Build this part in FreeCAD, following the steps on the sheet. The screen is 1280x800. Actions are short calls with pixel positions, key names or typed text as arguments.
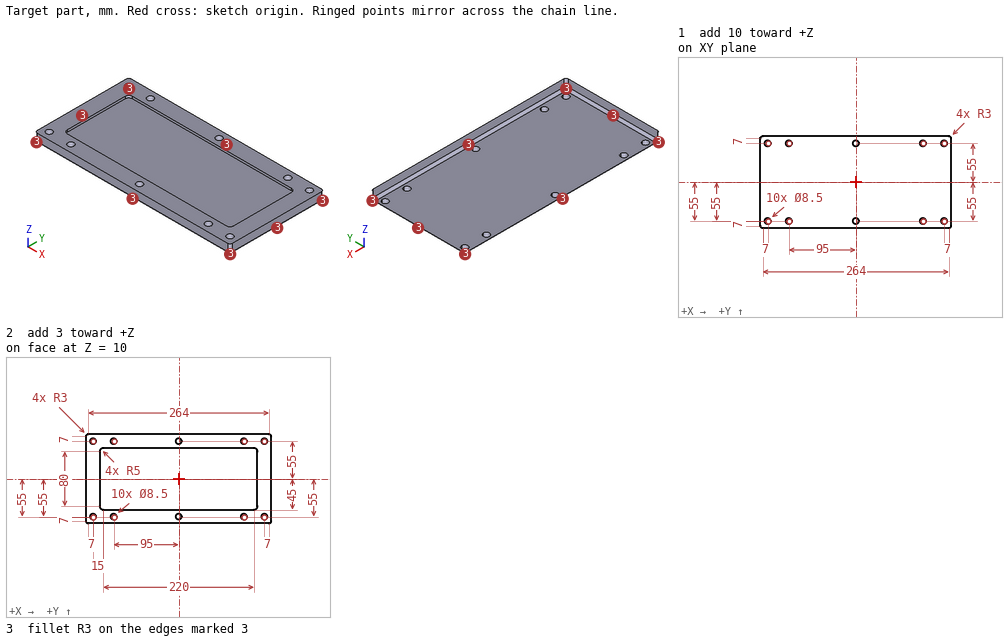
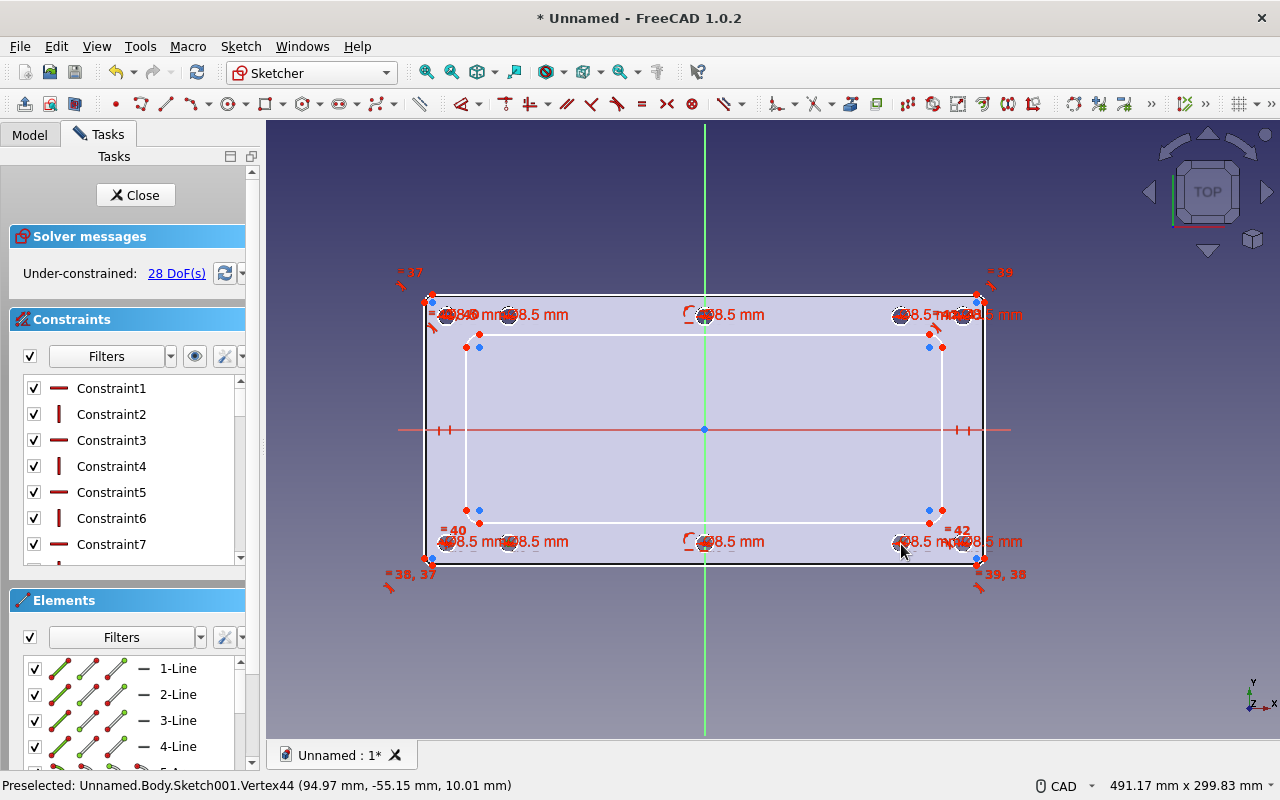
click(705, 671)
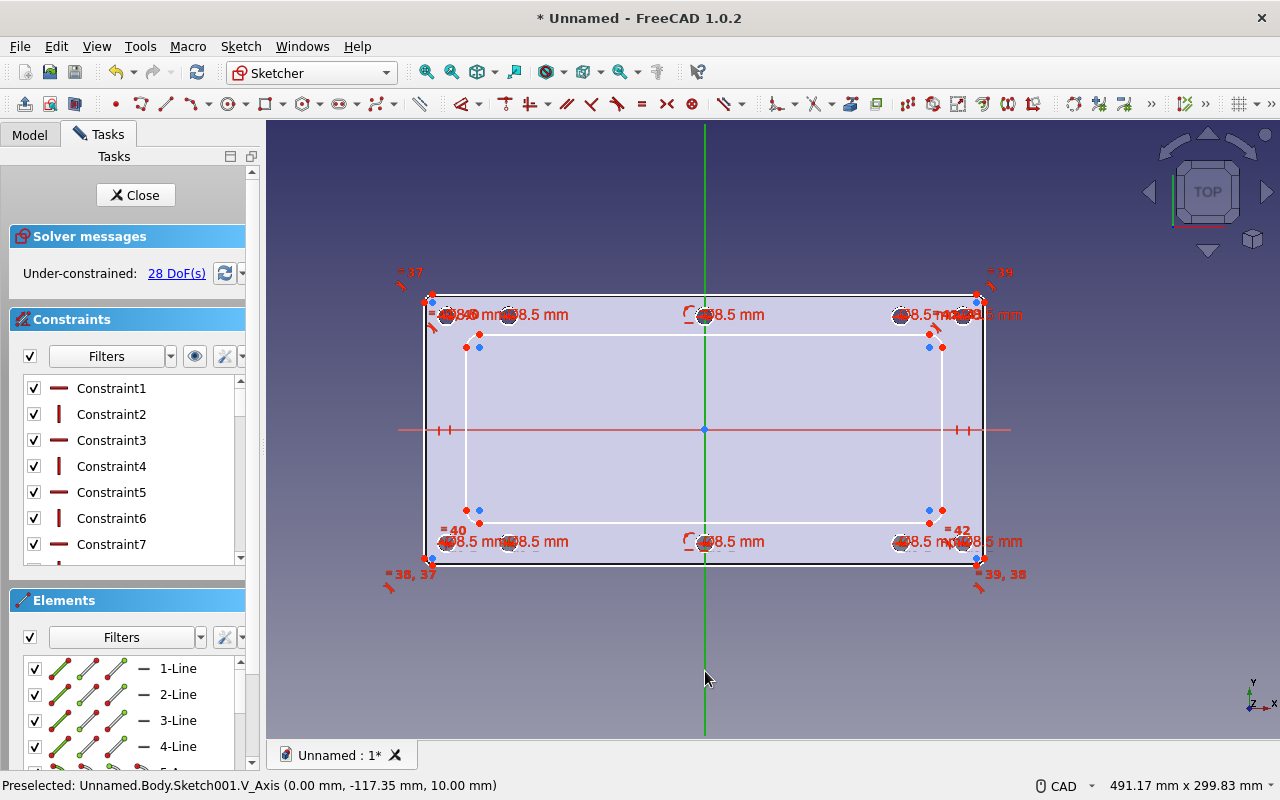
click(667, 104)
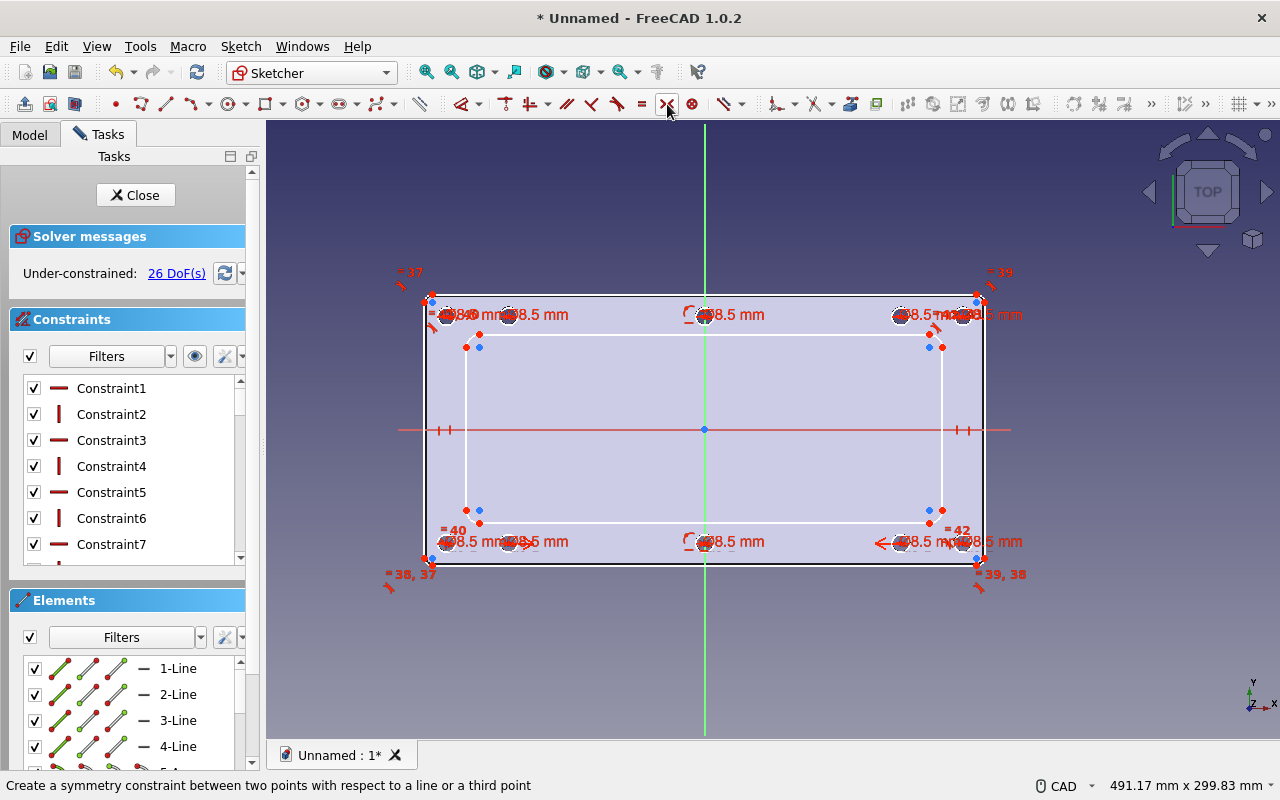
click(447, 544)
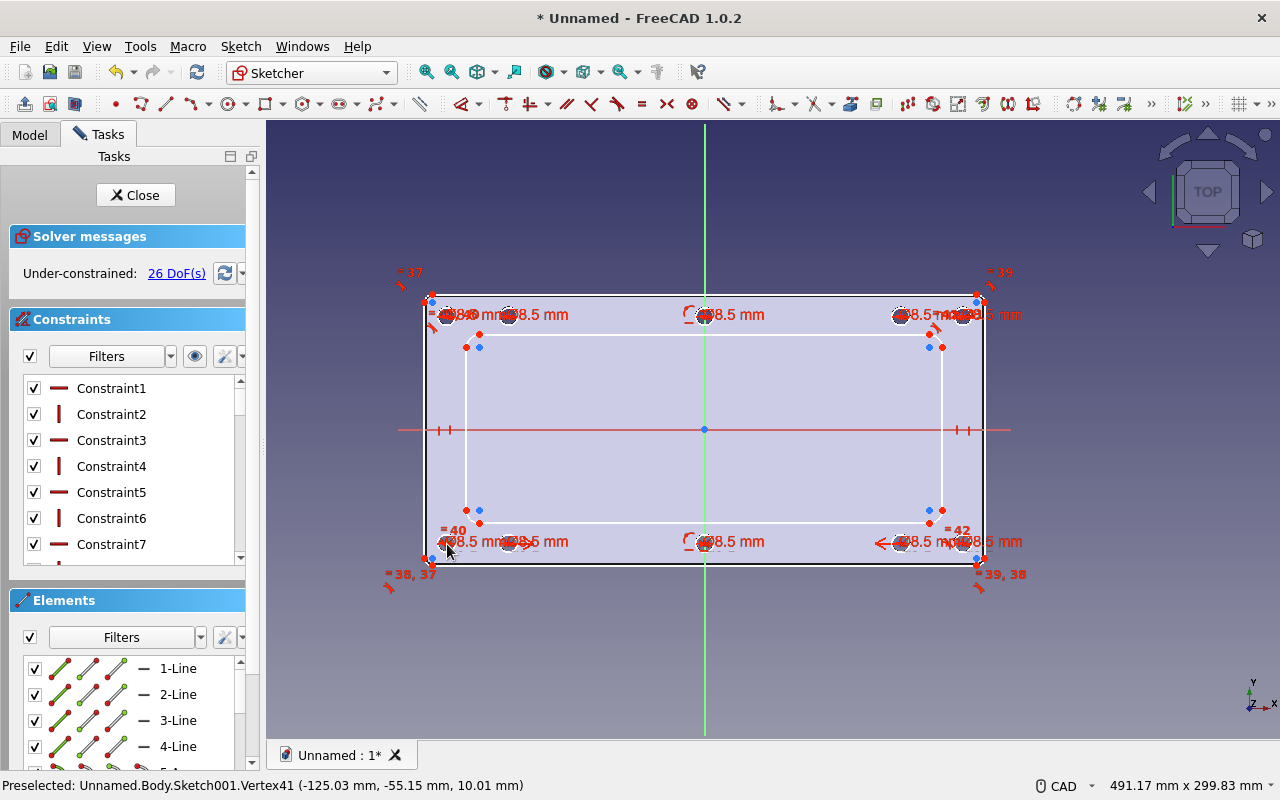
scroll(963, 544, up, 4)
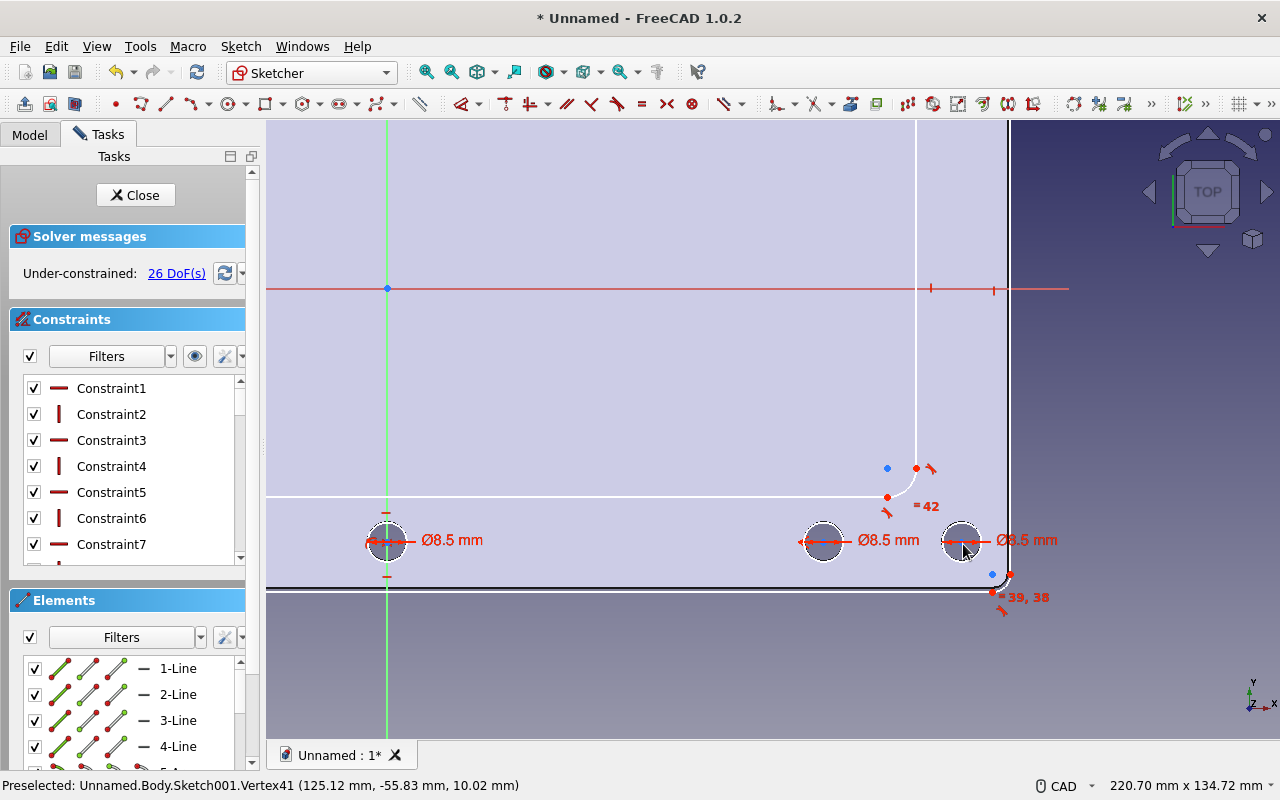
click(962, 542)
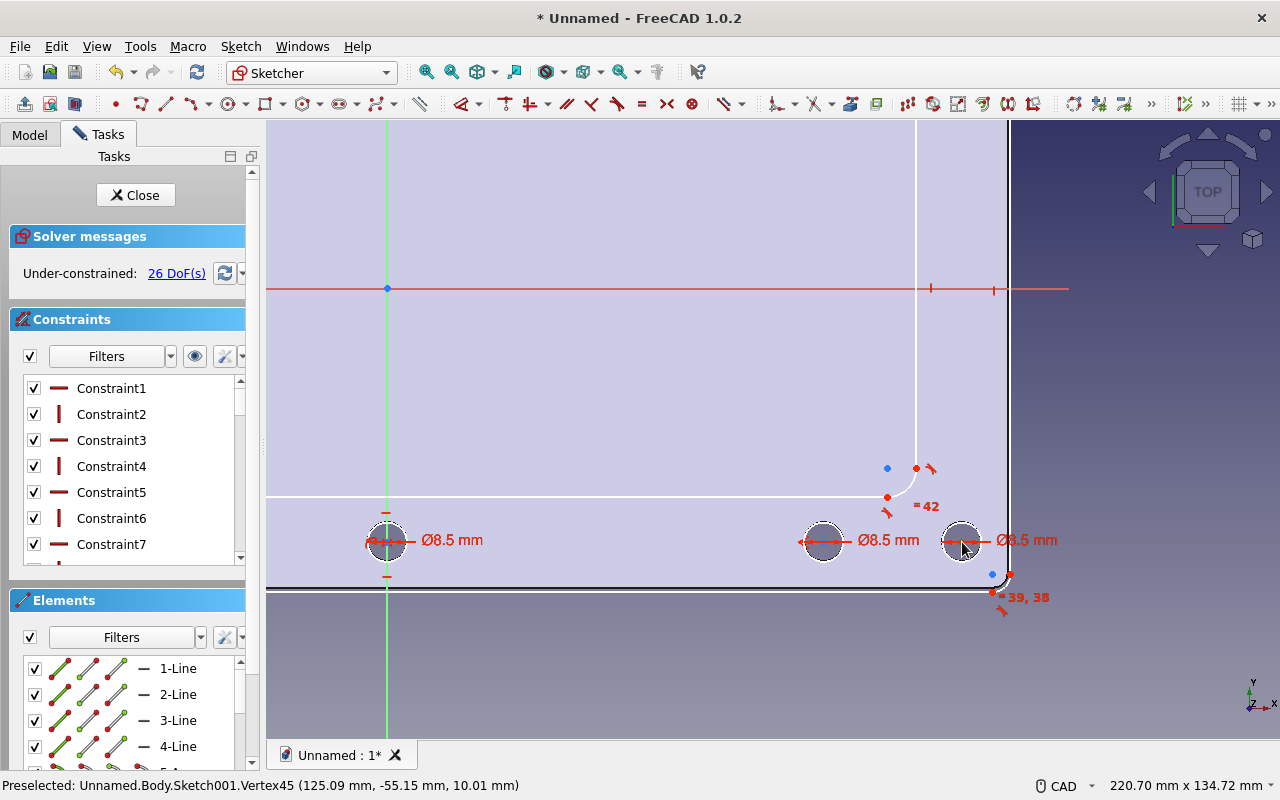
click(387, 671)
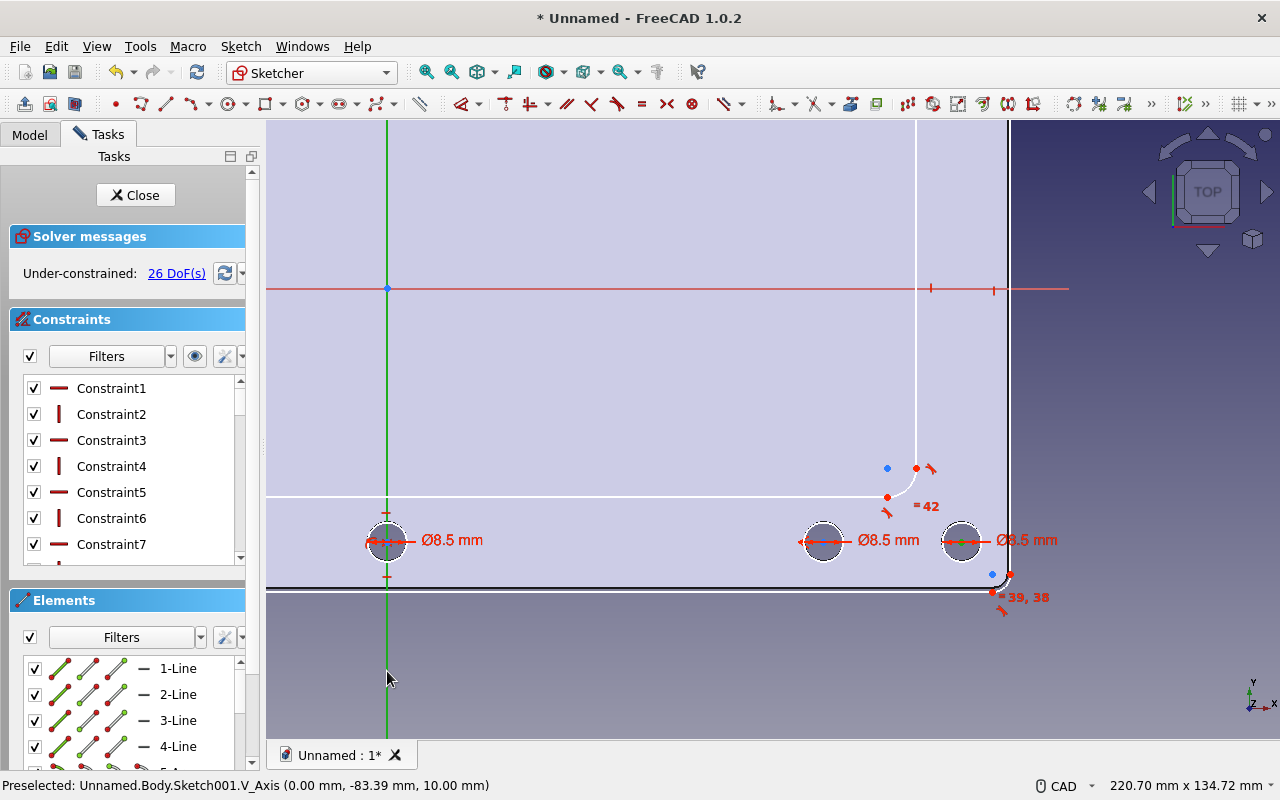
click(667, 104)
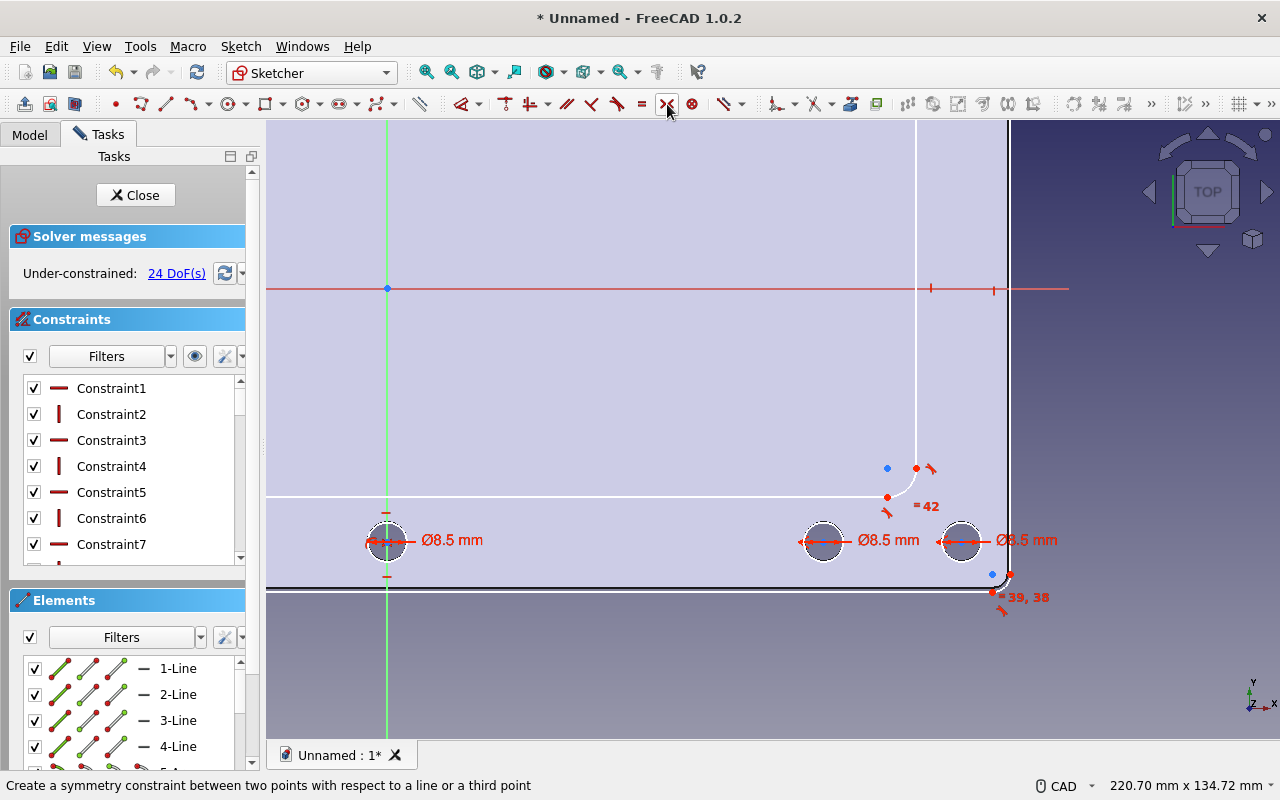
scroll(963, 544, down, 4)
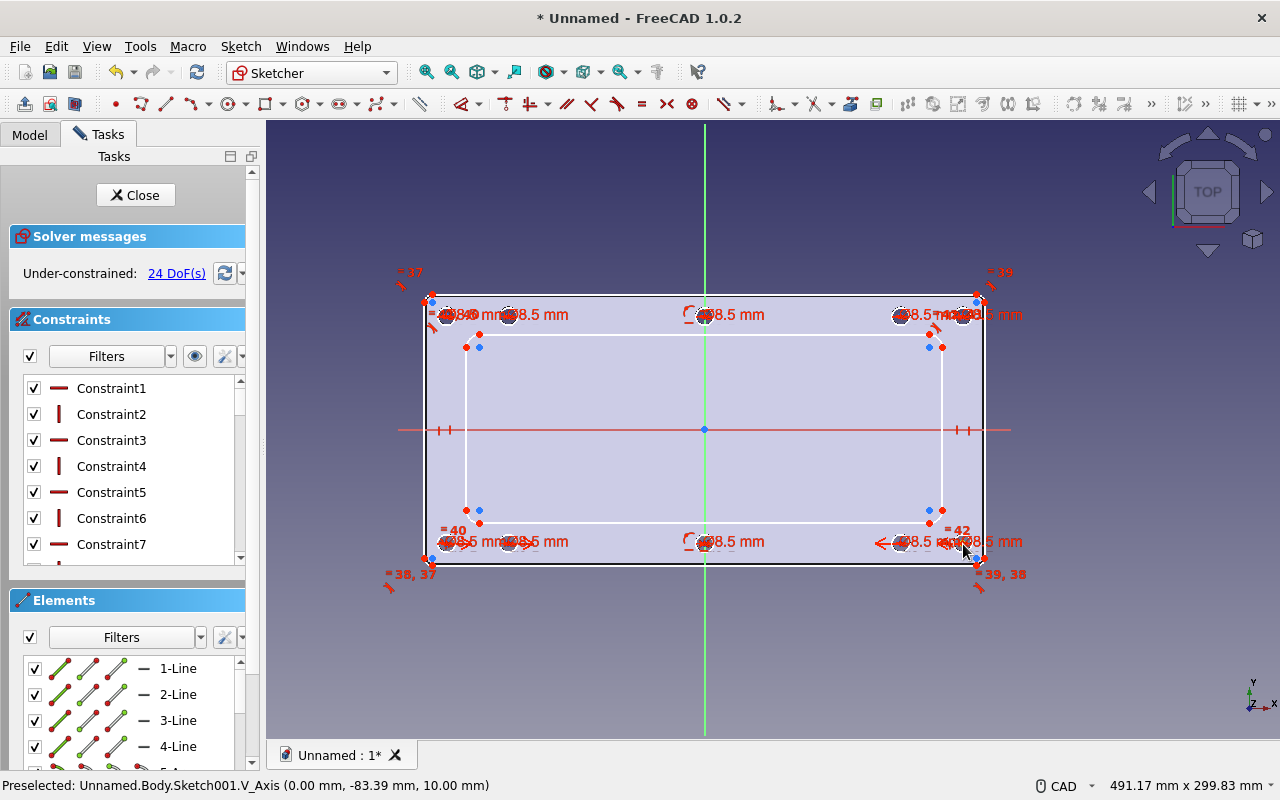
click(447, 544)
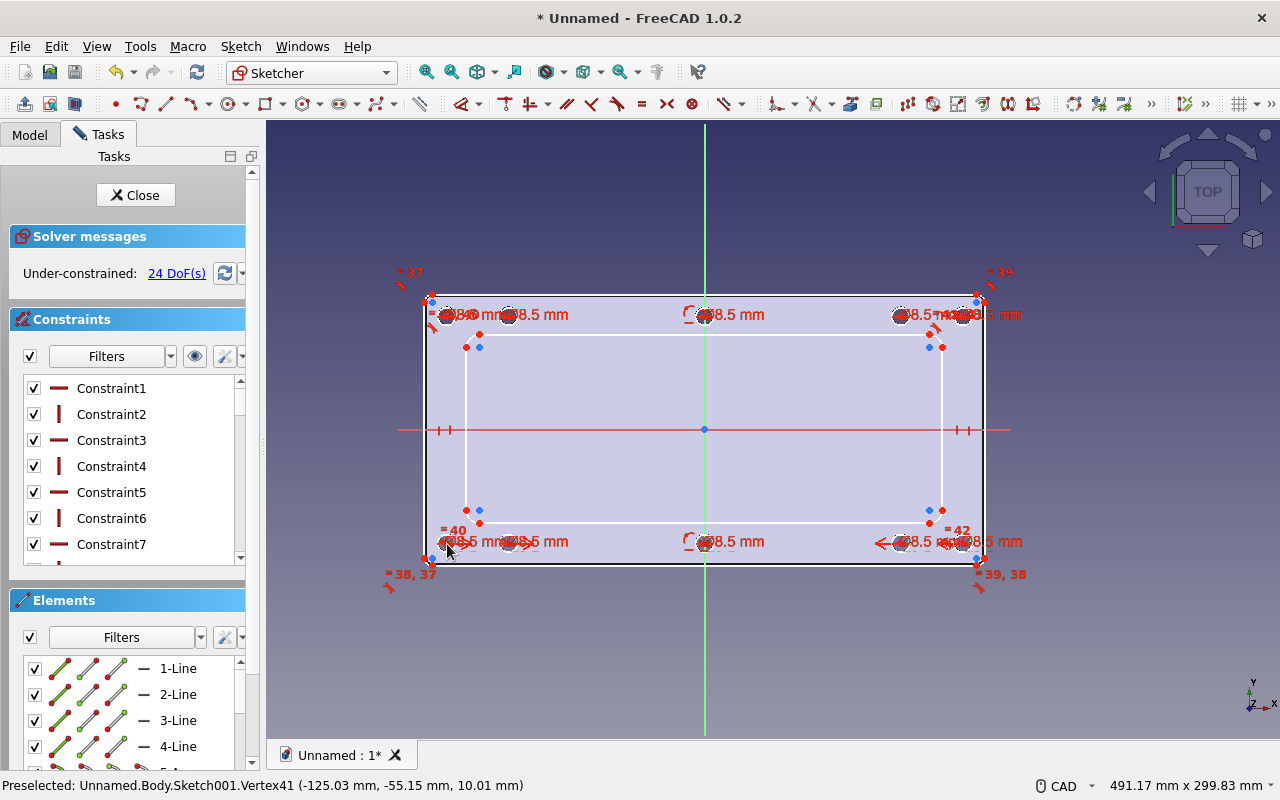
click(446, 317)